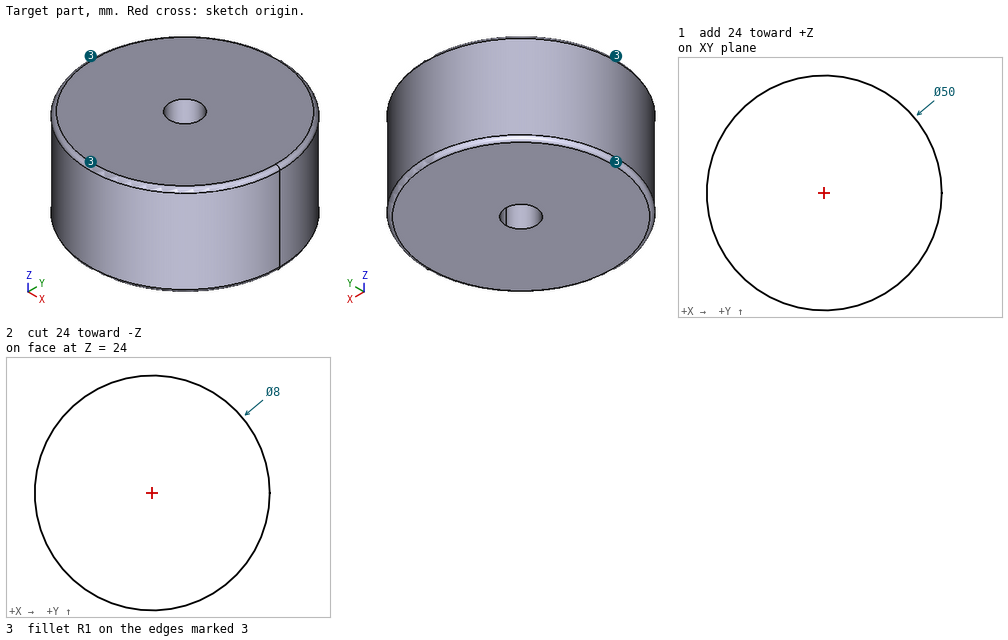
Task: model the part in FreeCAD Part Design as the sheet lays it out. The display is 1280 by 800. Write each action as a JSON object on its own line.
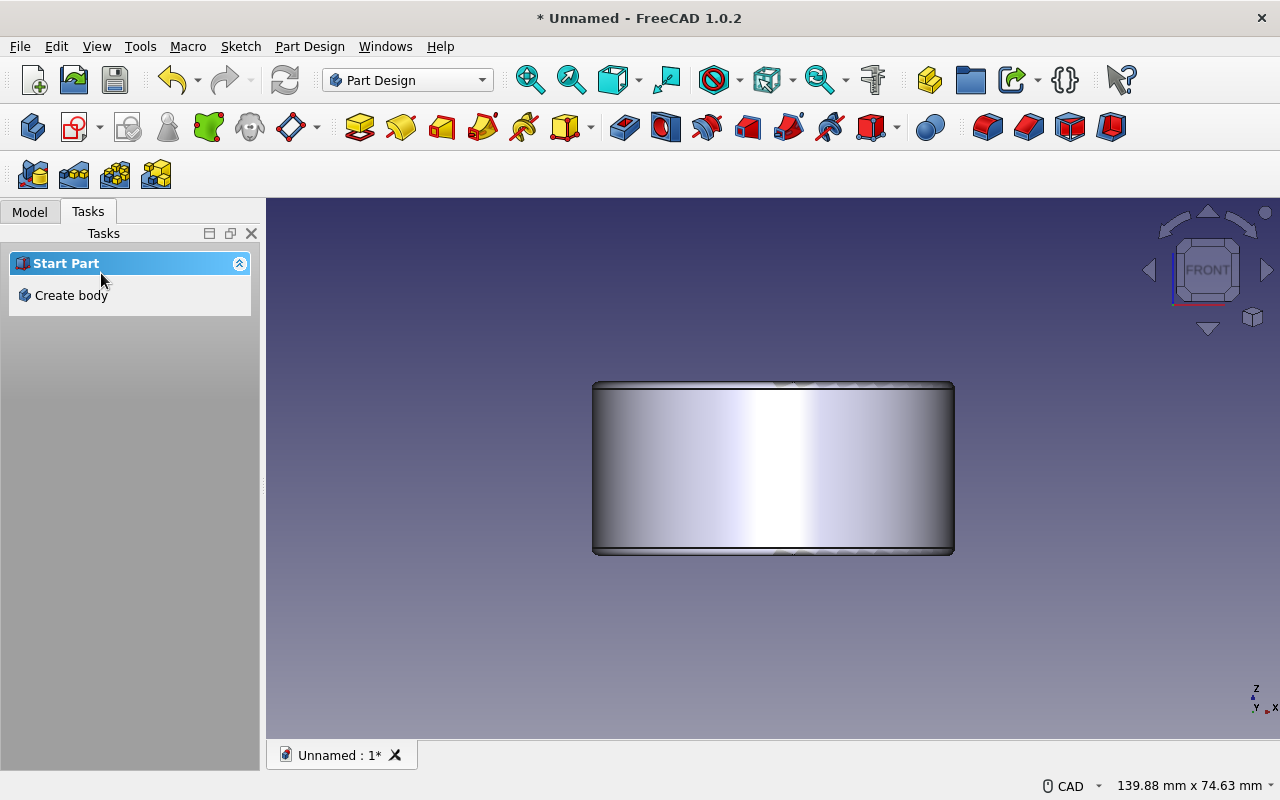
{"action": "key", "text": "0"}